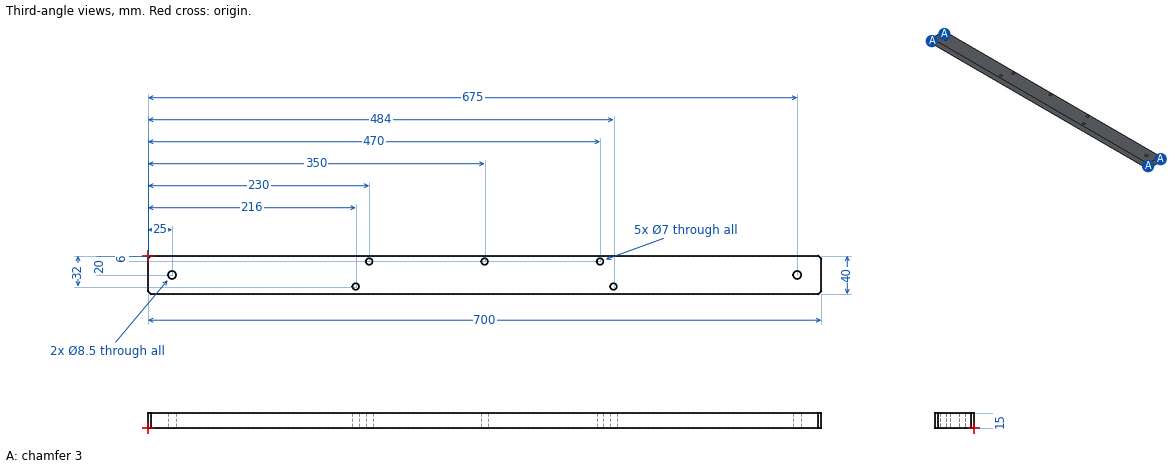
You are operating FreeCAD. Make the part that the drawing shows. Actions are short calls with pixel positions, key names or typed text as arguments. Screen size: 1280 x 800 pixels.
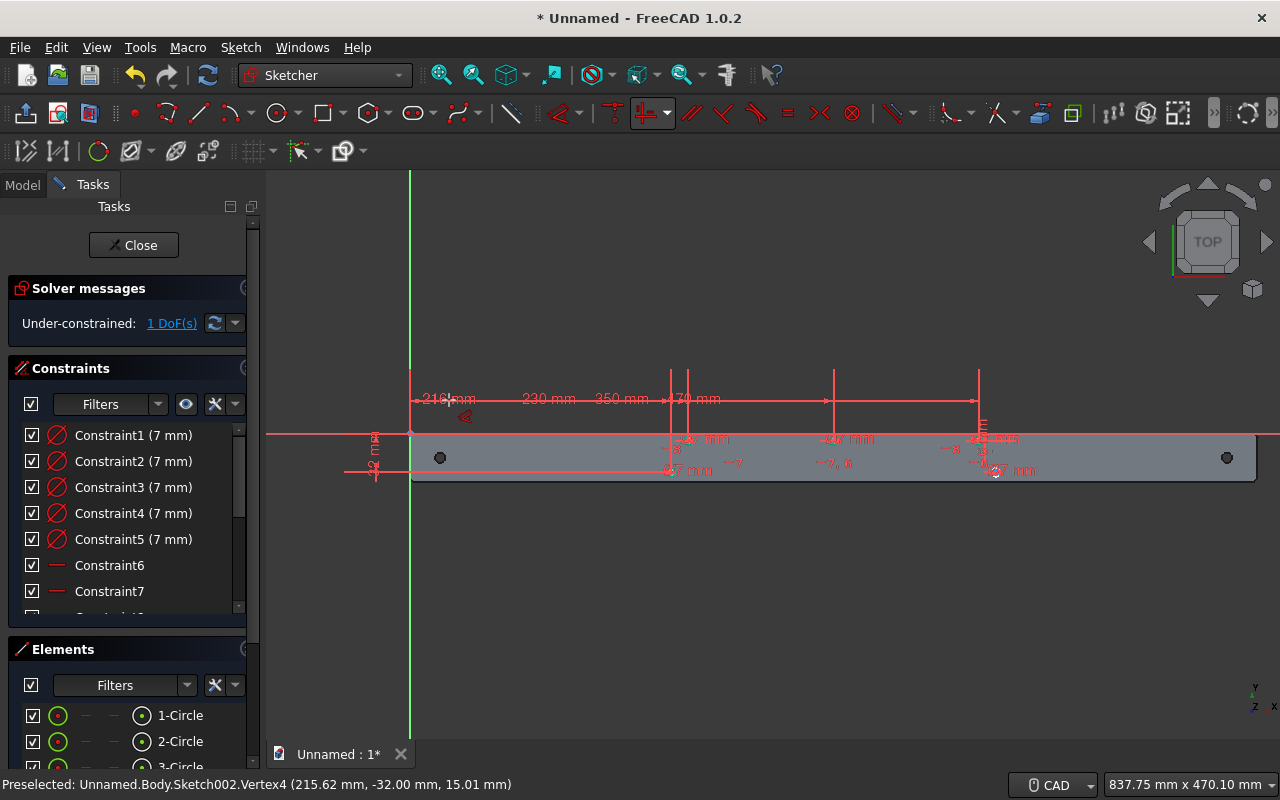
click(996, 472)
click(838, 400)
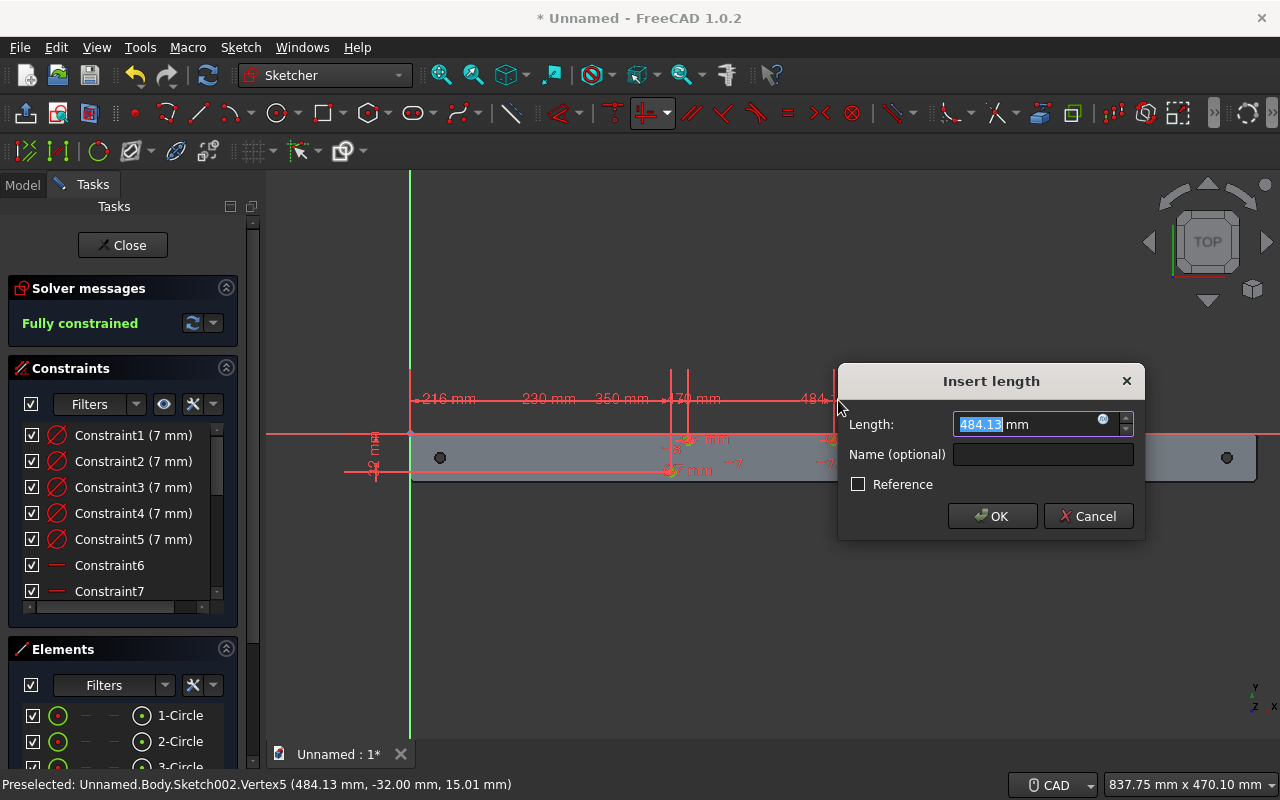
text(484)
key(Return)
key(Escape)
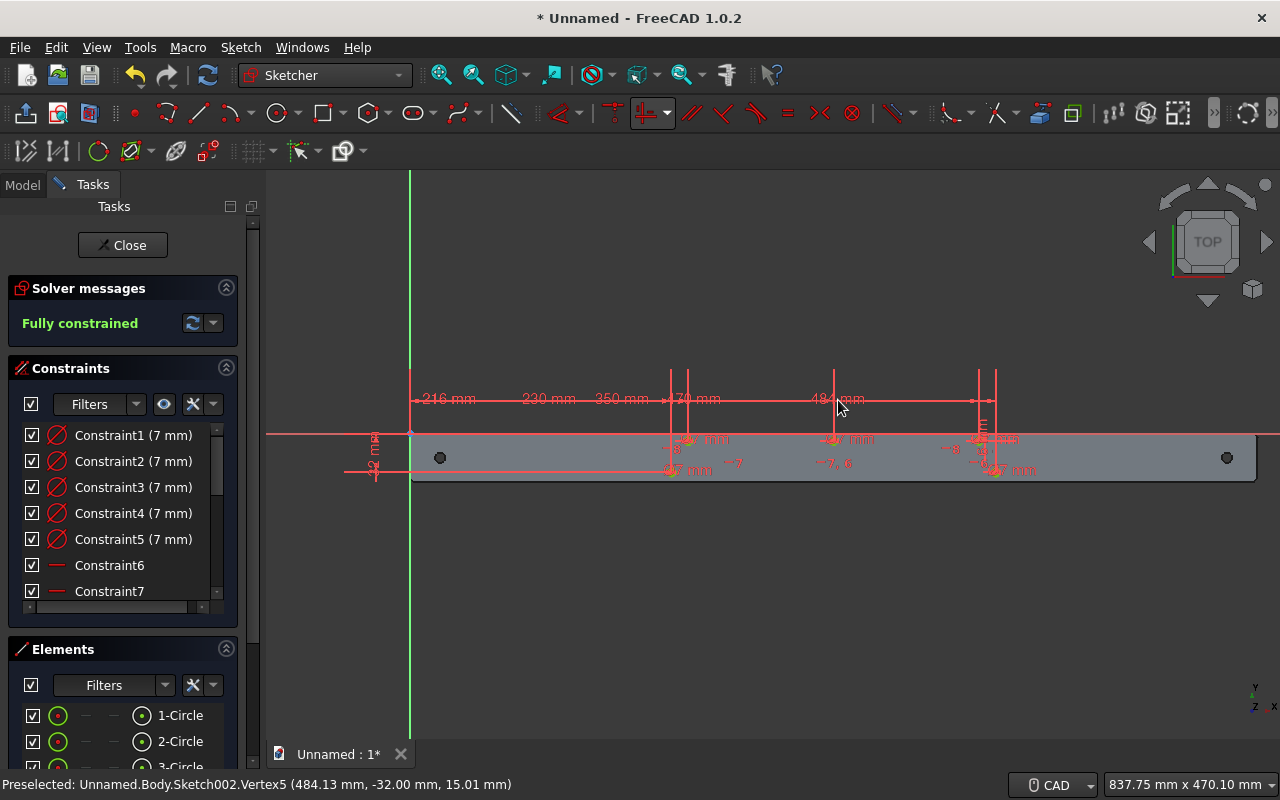
click(123, 245)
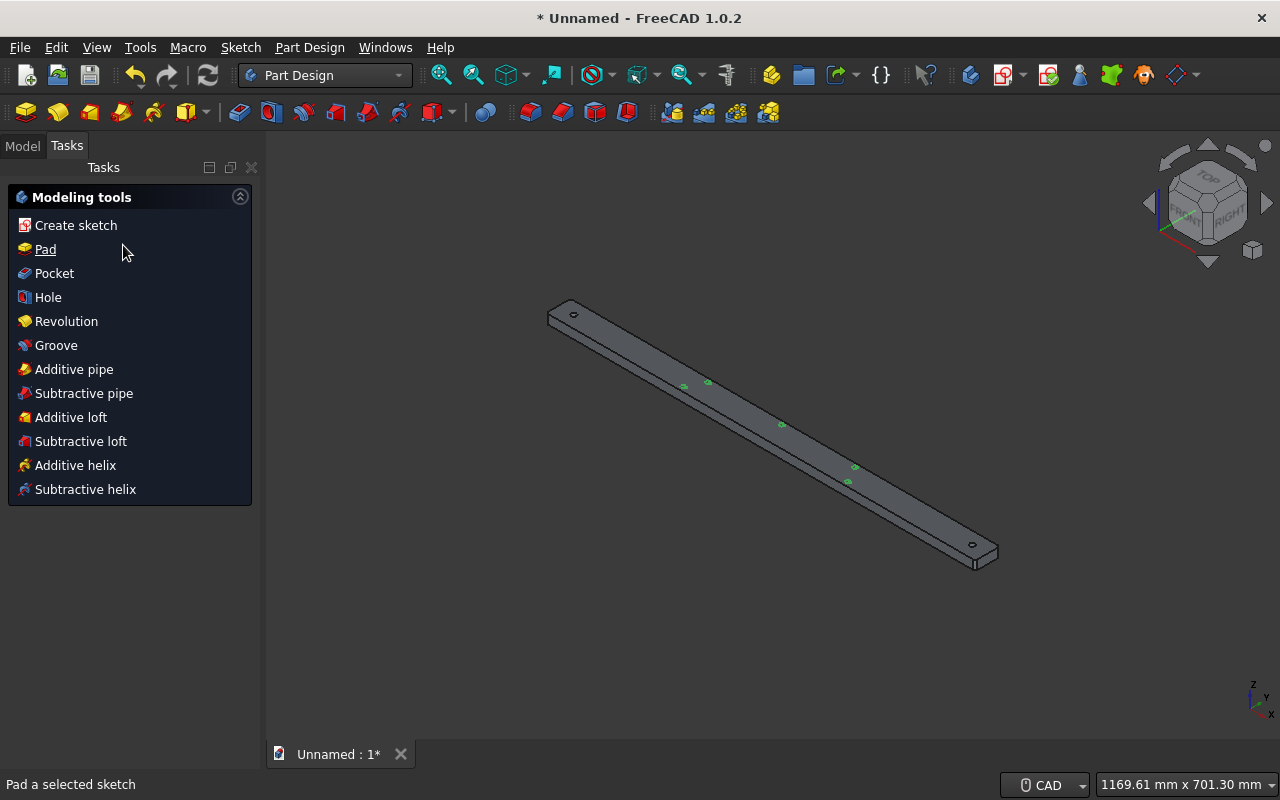
click(272, 112)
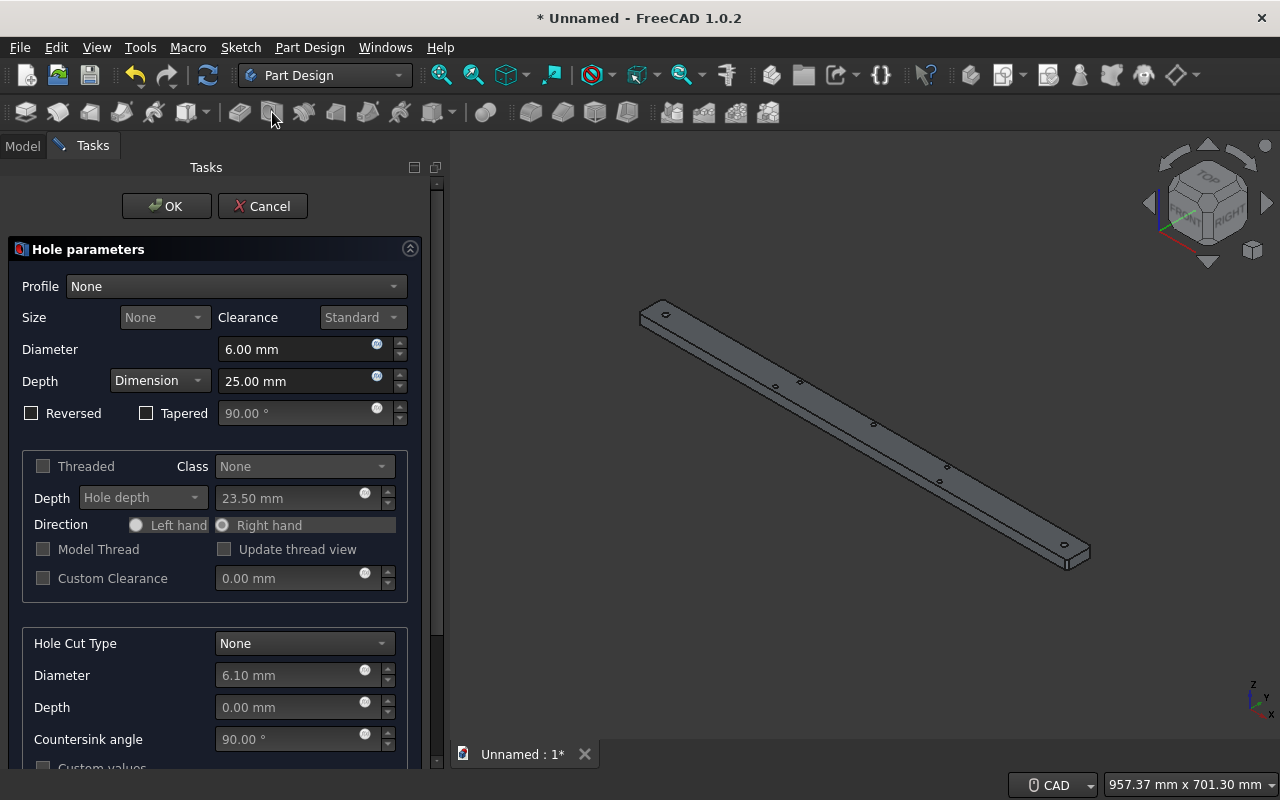
triple_click(305, 349)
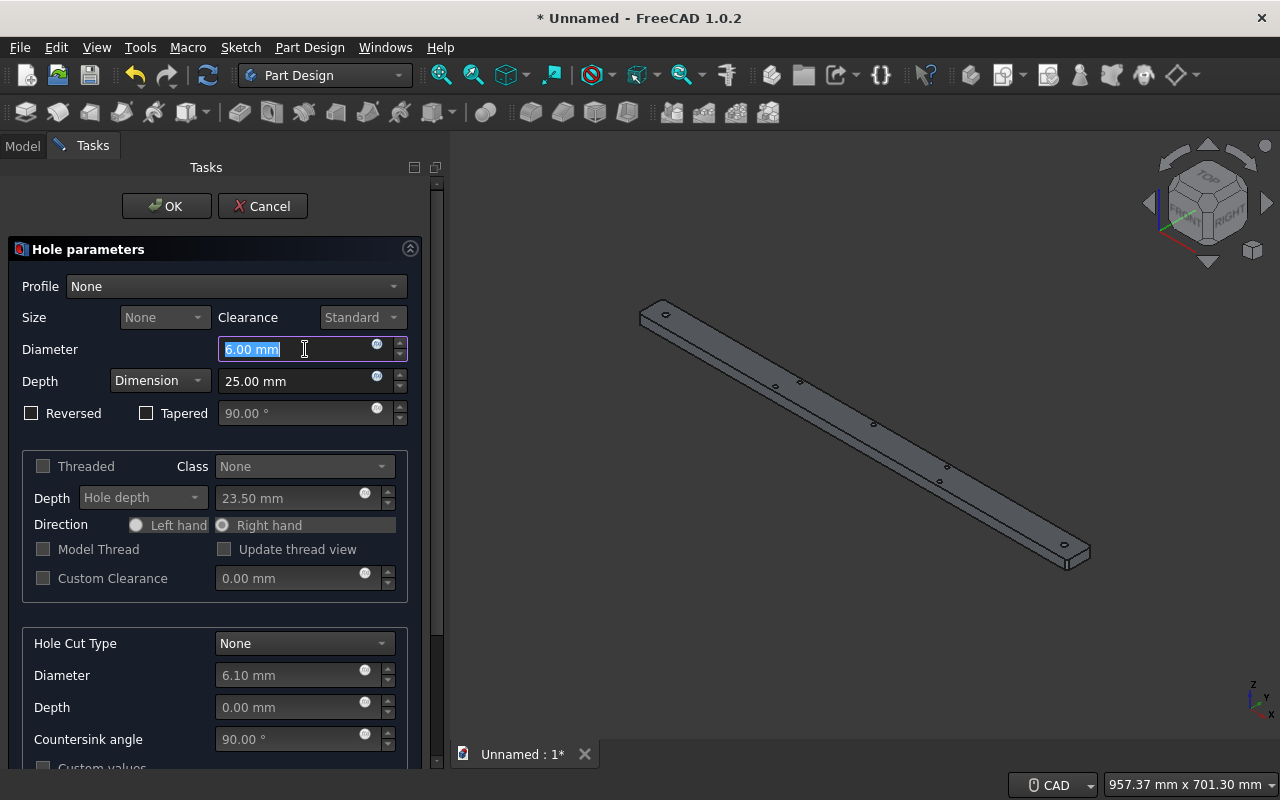
text(7)
key(Tab)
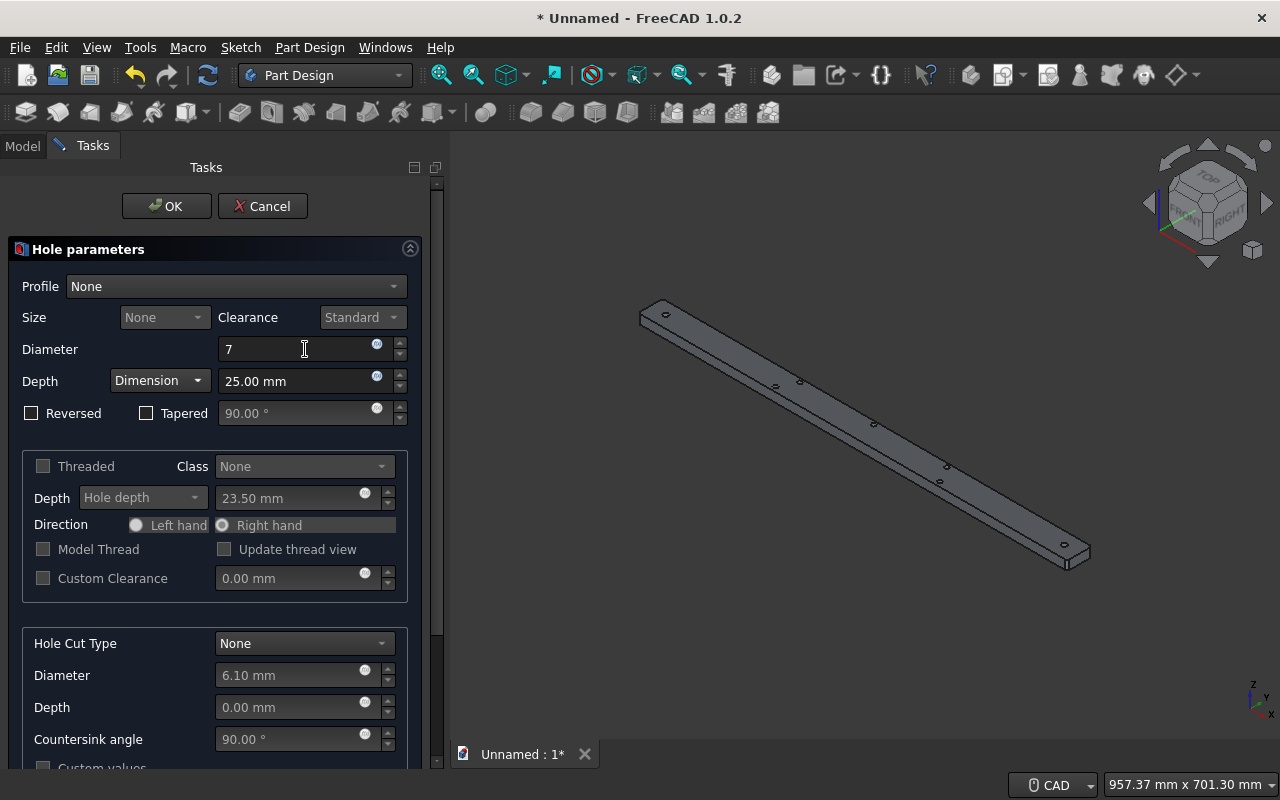
click(161, 380)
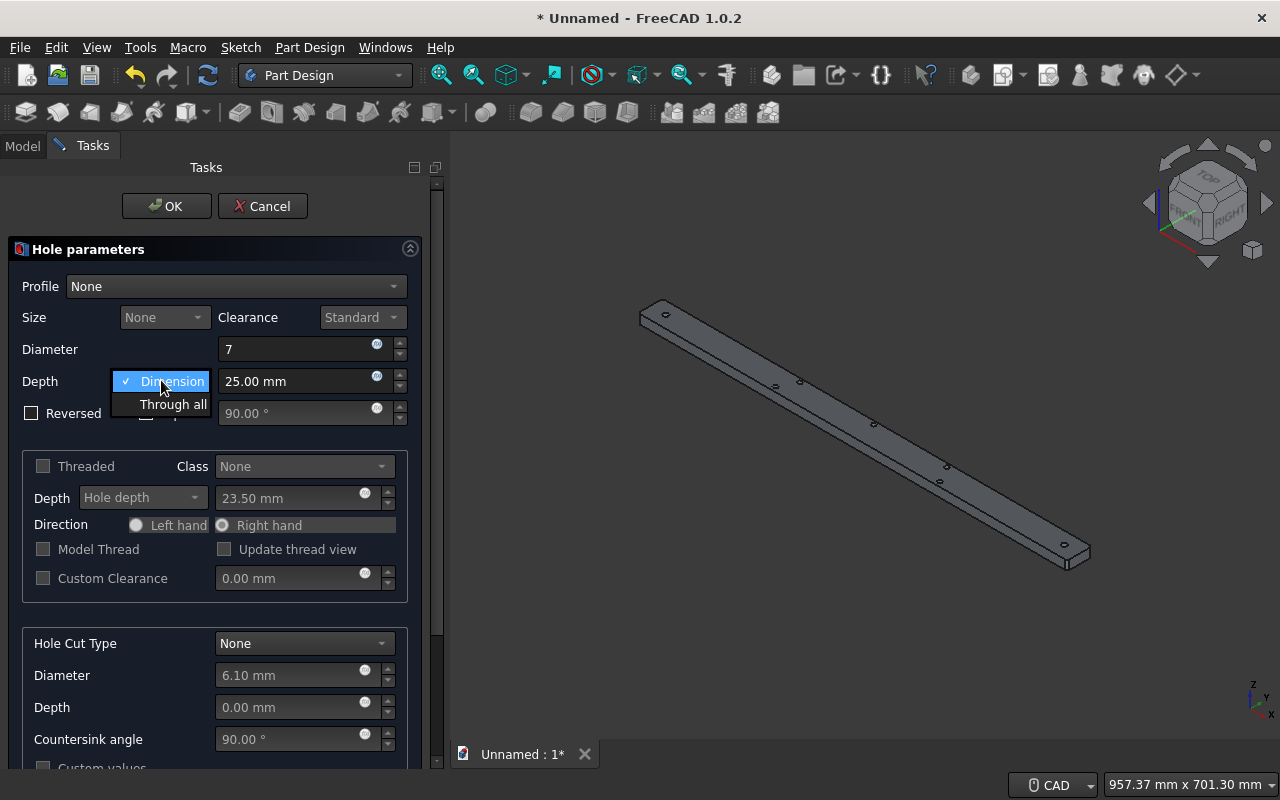
click(160, 404)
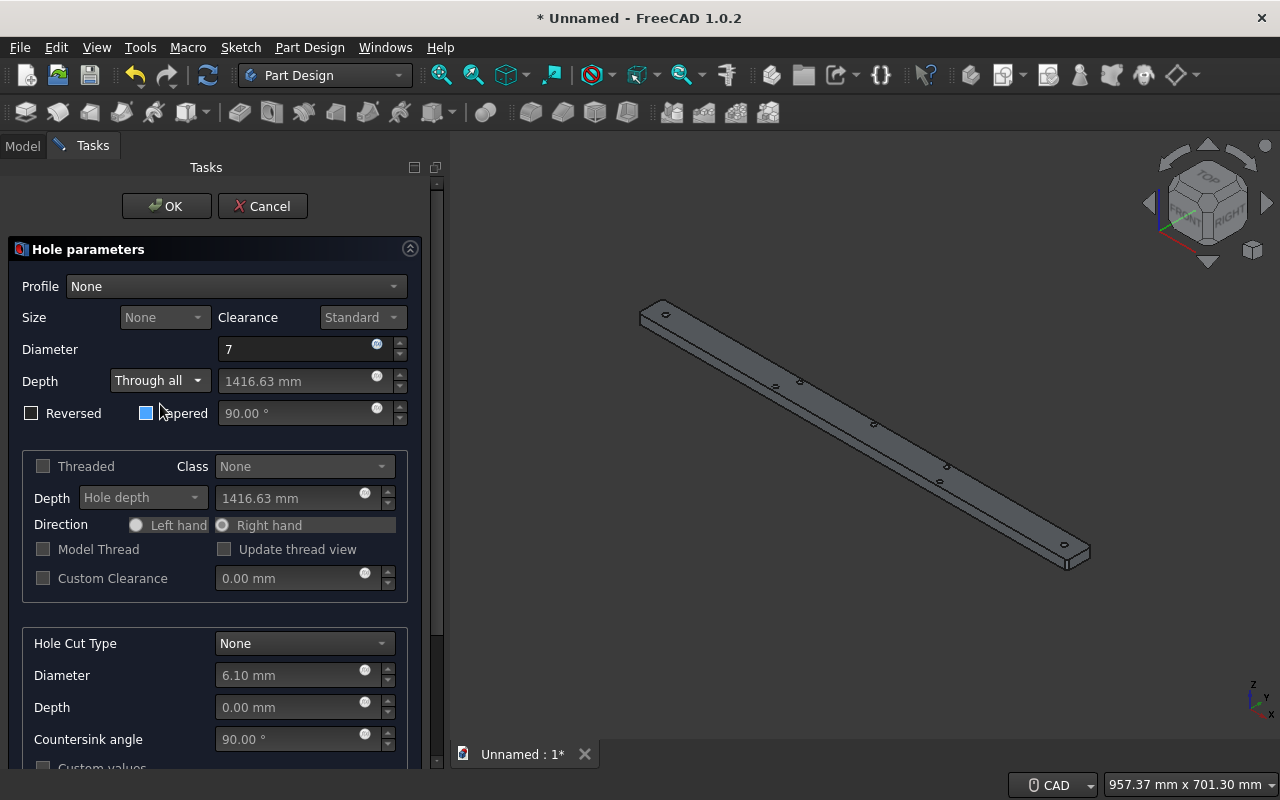
click(167, 206)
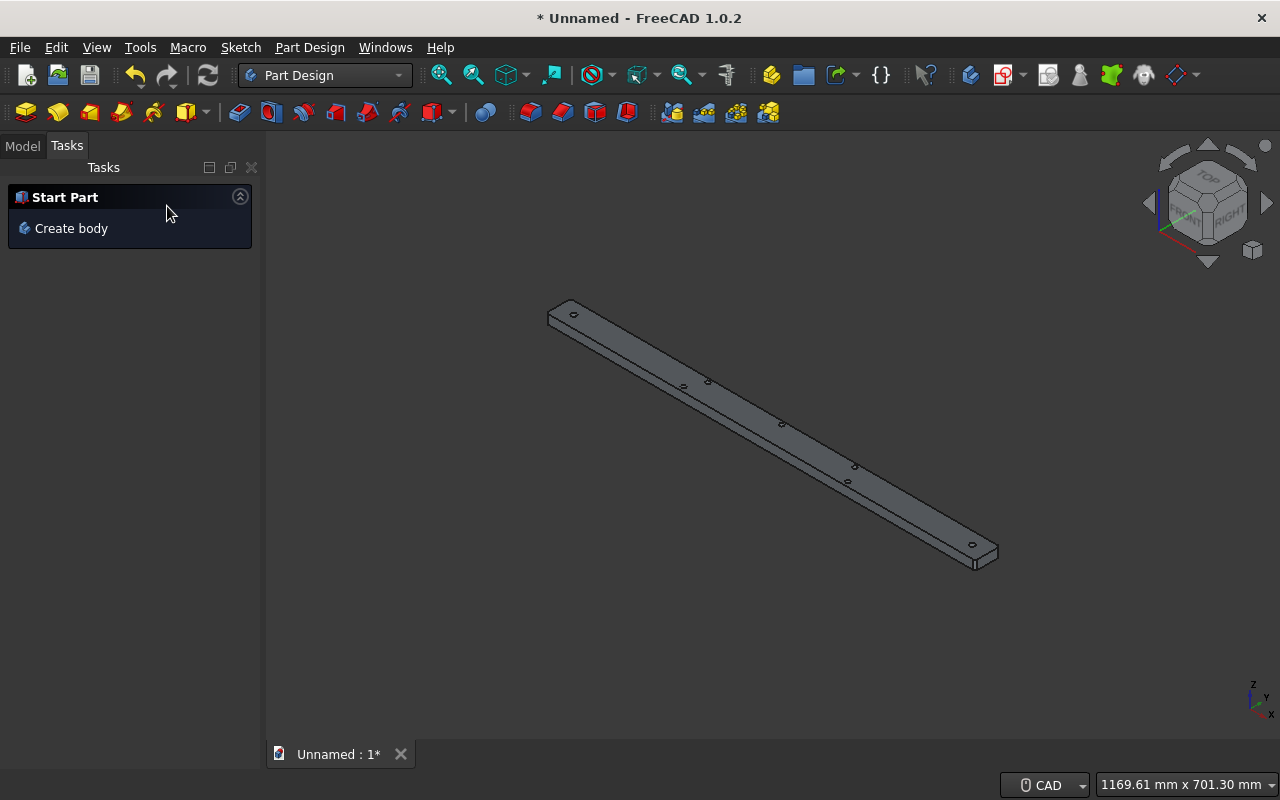
click(442, 76)